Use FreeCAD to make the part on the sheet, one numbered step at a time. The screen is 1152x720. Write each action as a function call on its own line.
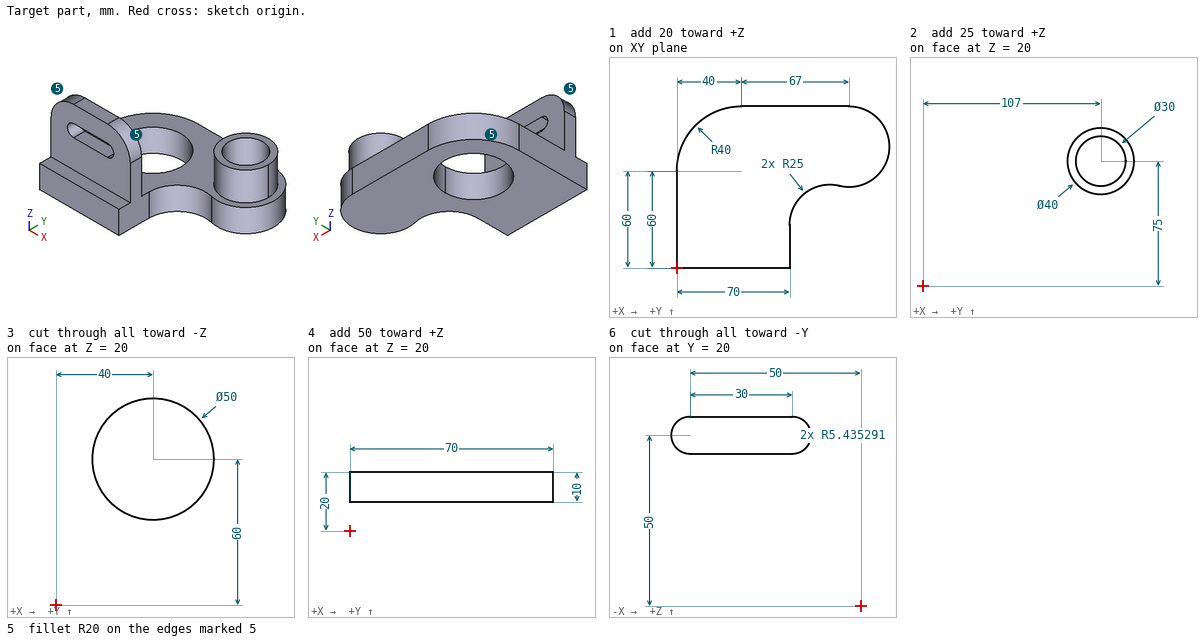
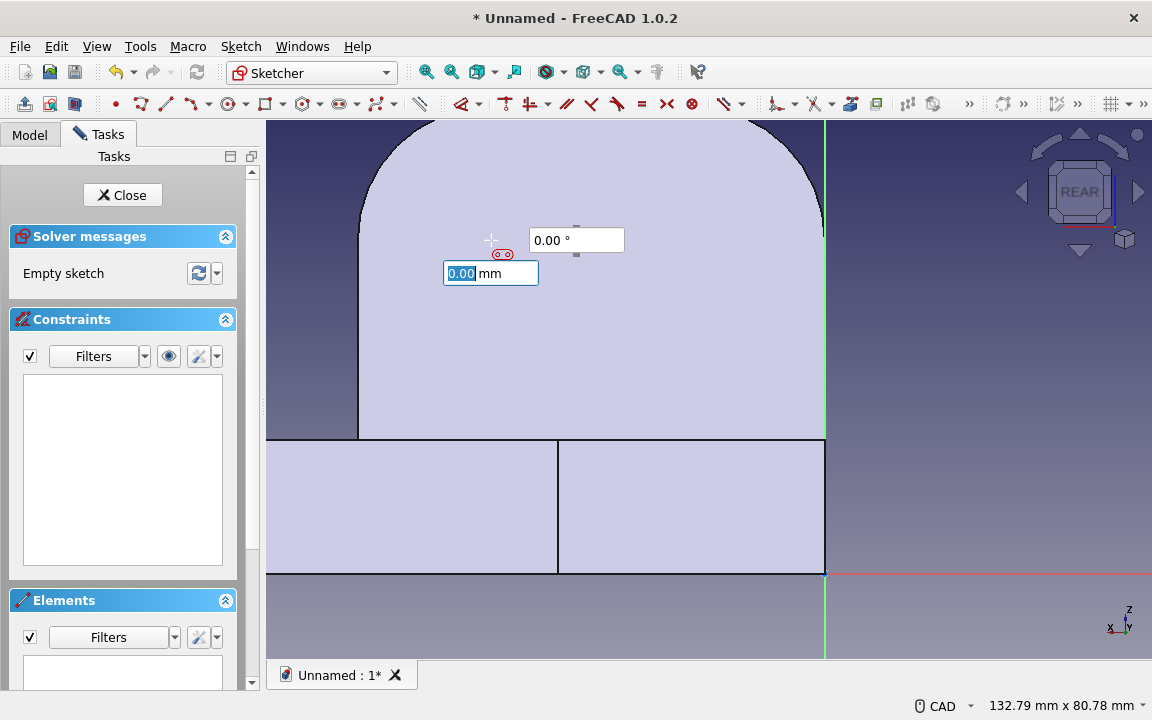
click(691, 240)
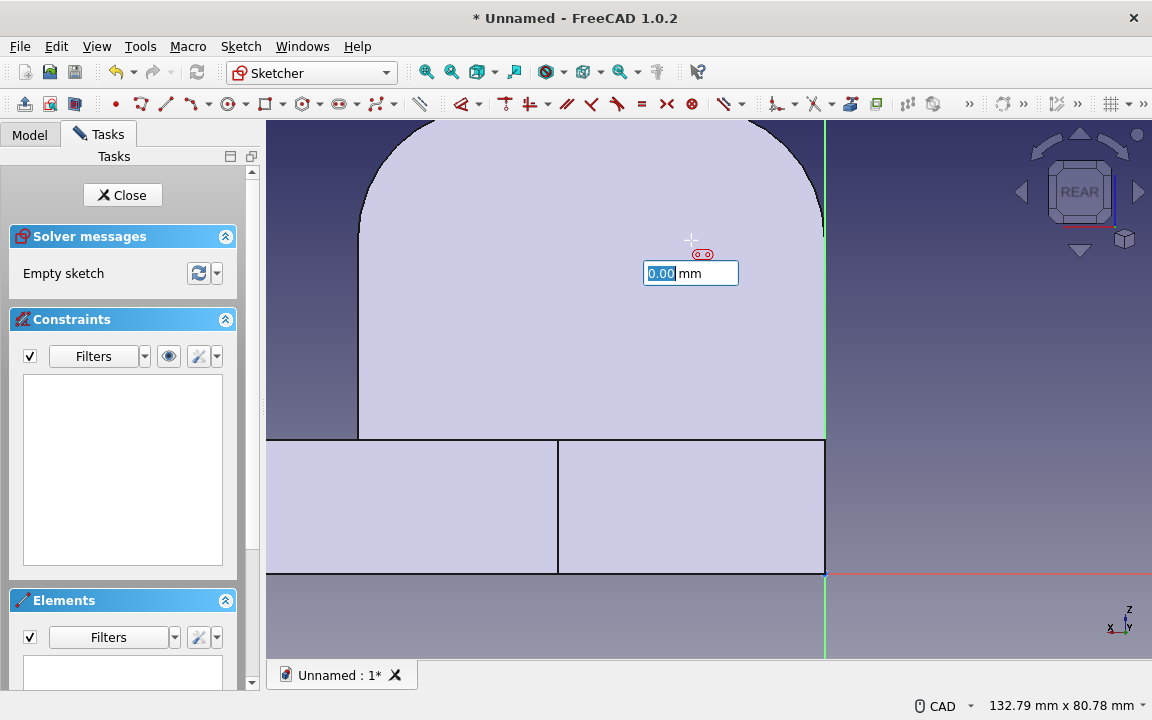
click(591, 277)
key(Escape)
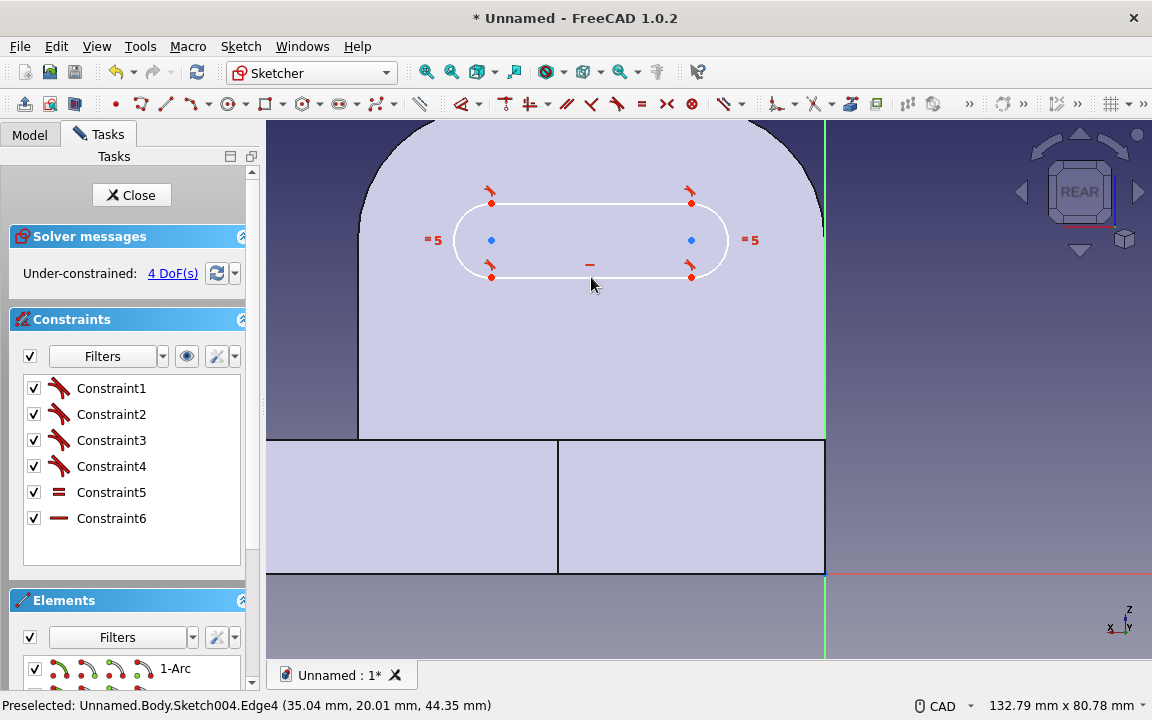
click(460, 104)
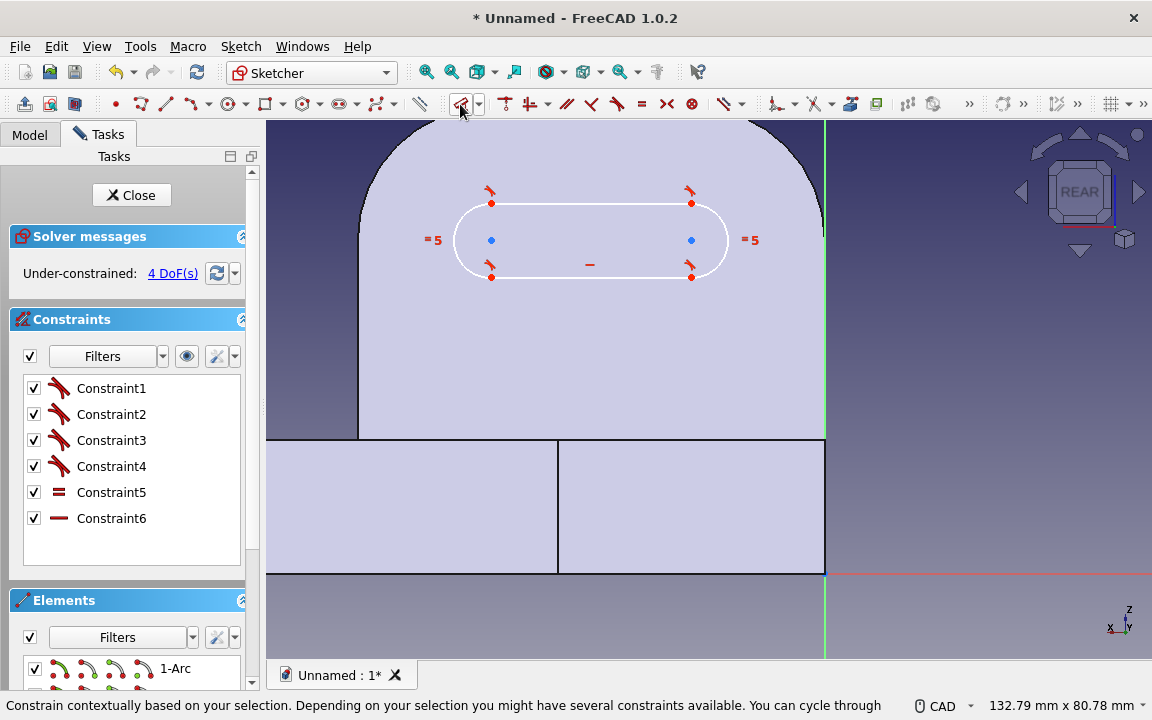
click(461, 219)
click(435, 200)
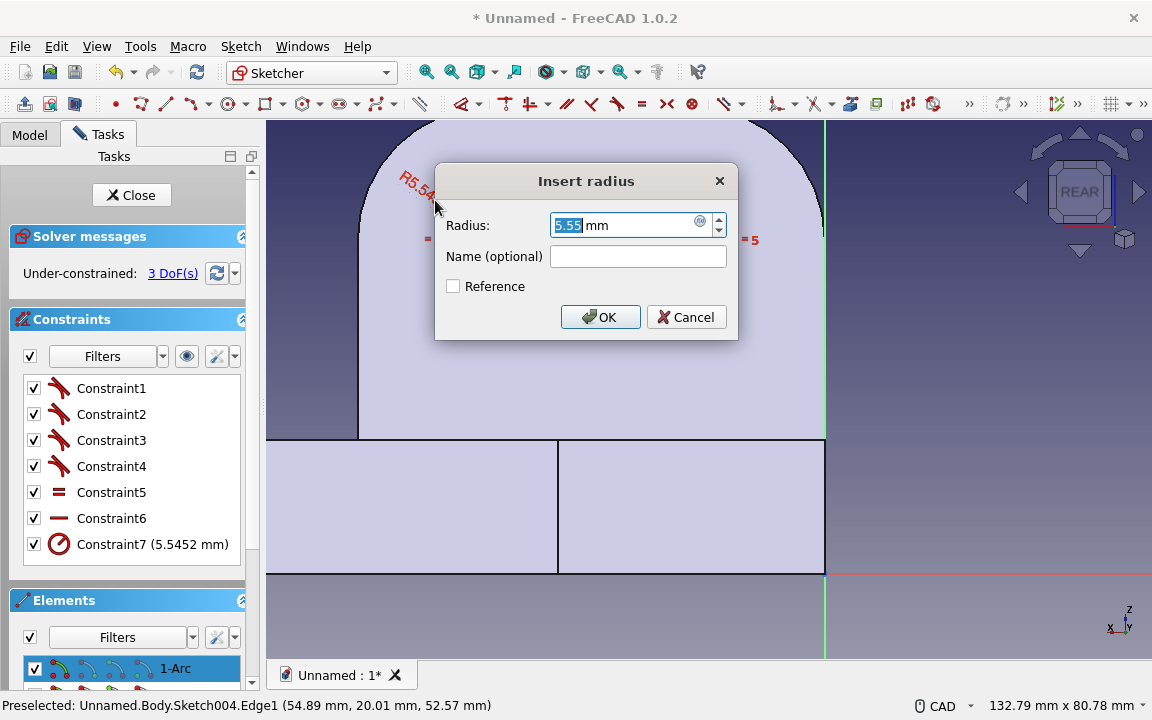
text(5.435291)
key(Return)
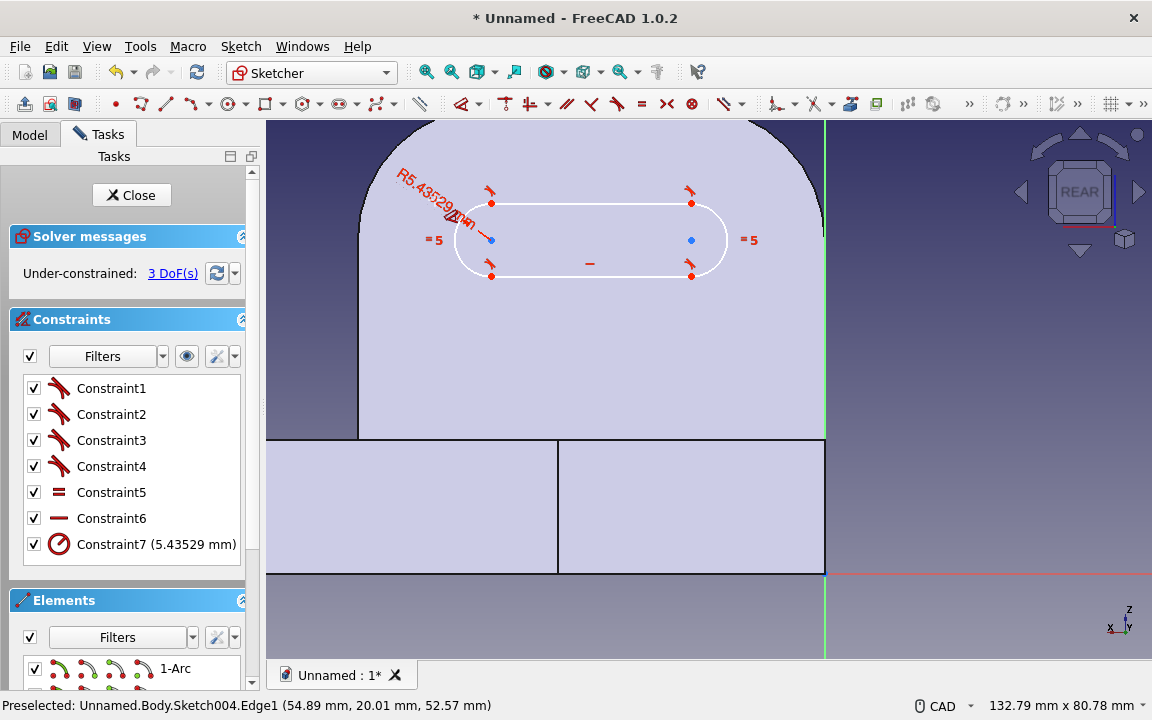
click(551, 204)
click(591, 170)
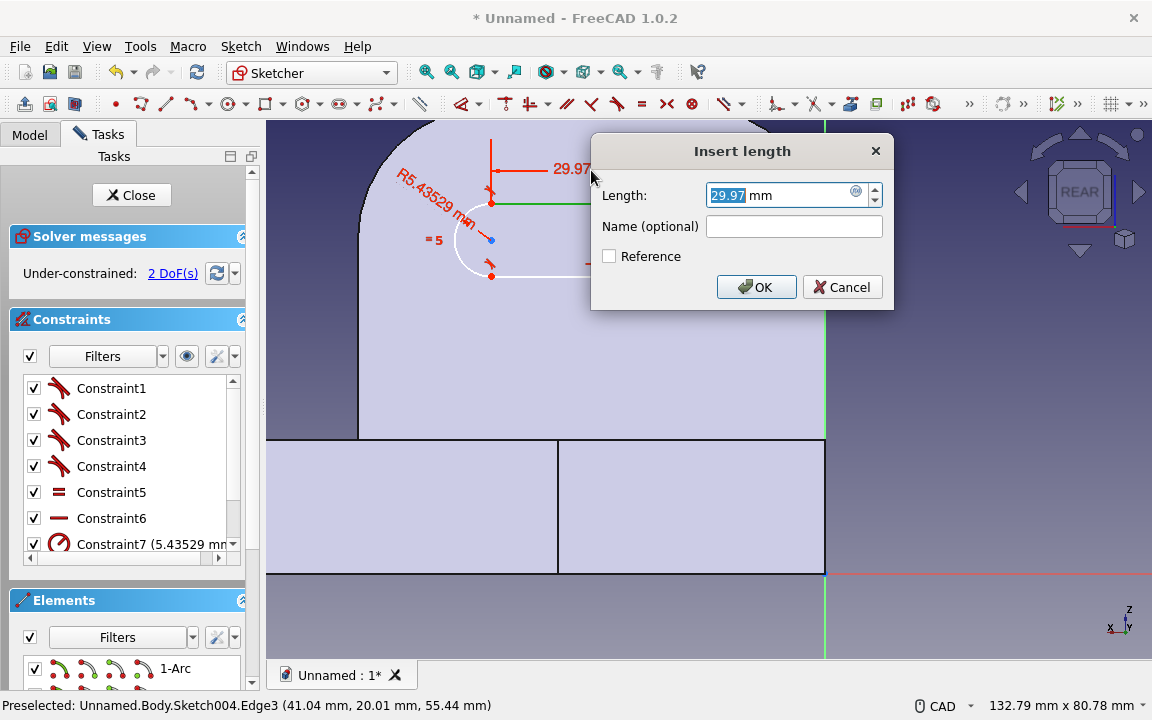
text(30)
key(Return)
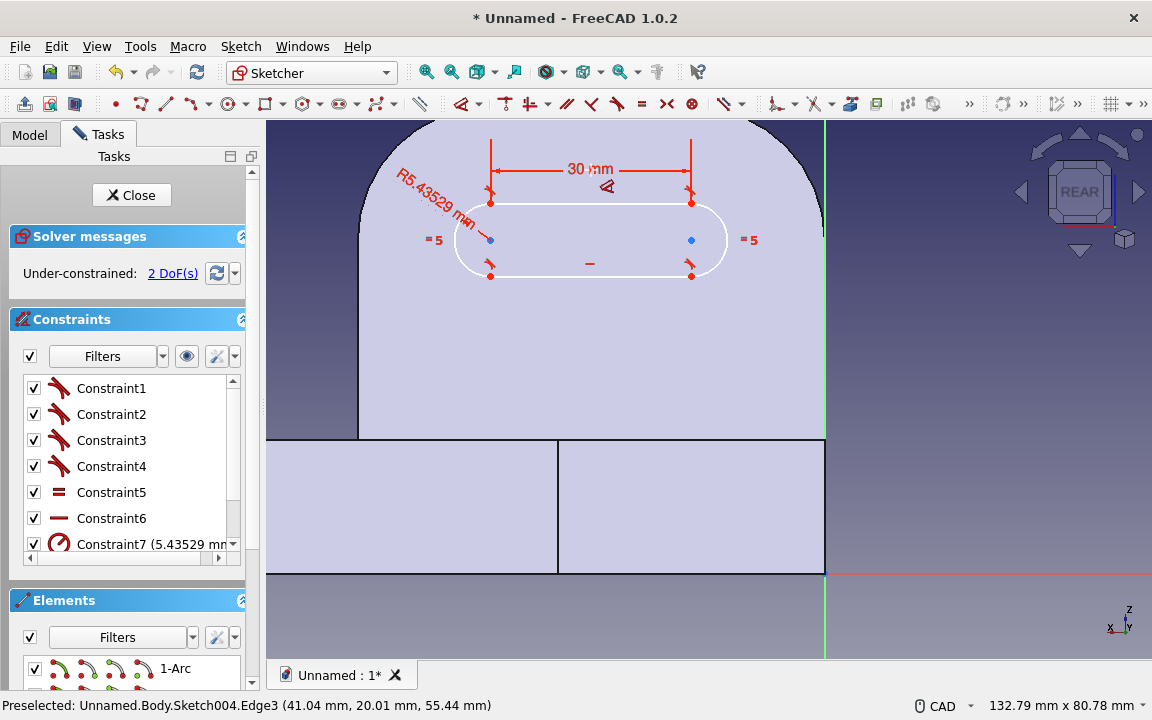
click(491, 204)
click(735, 170)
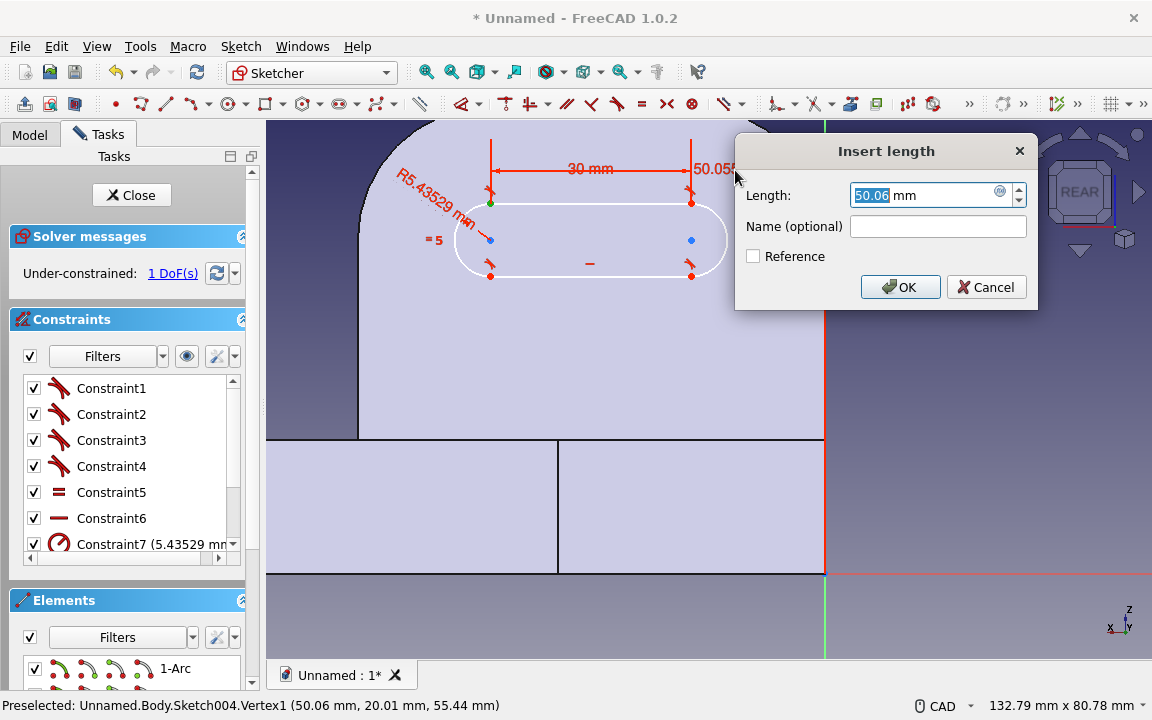
text(50)
key(Return)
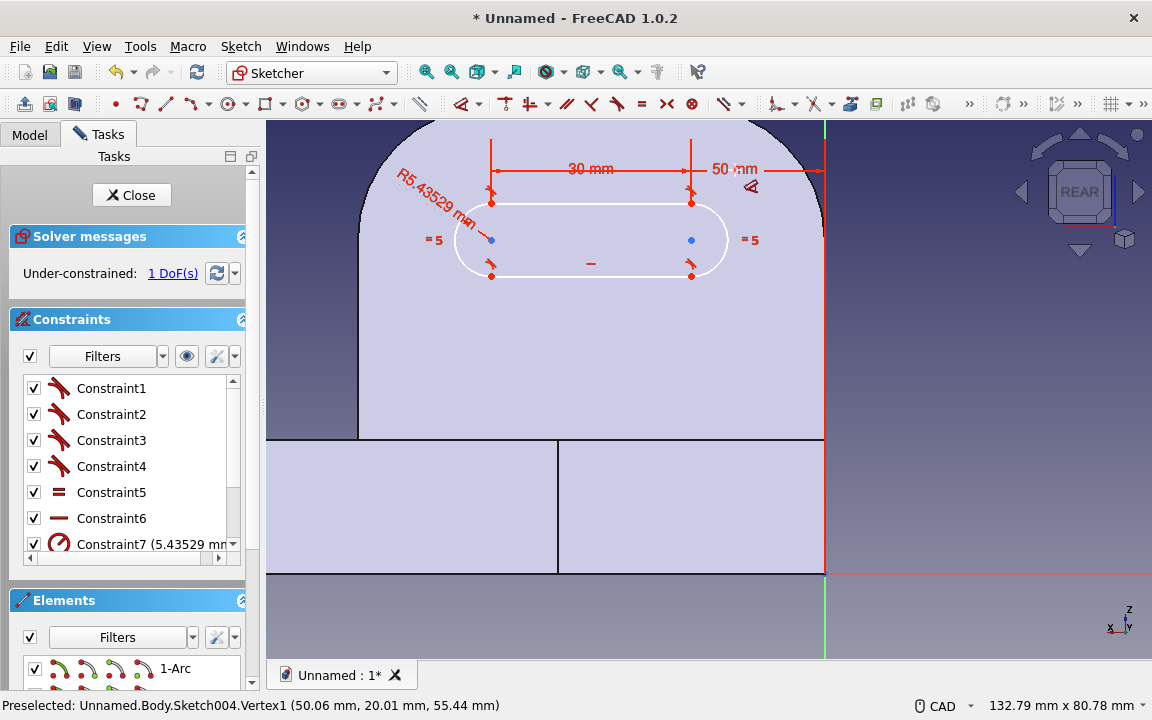
click(491, 240)
click(859, 407)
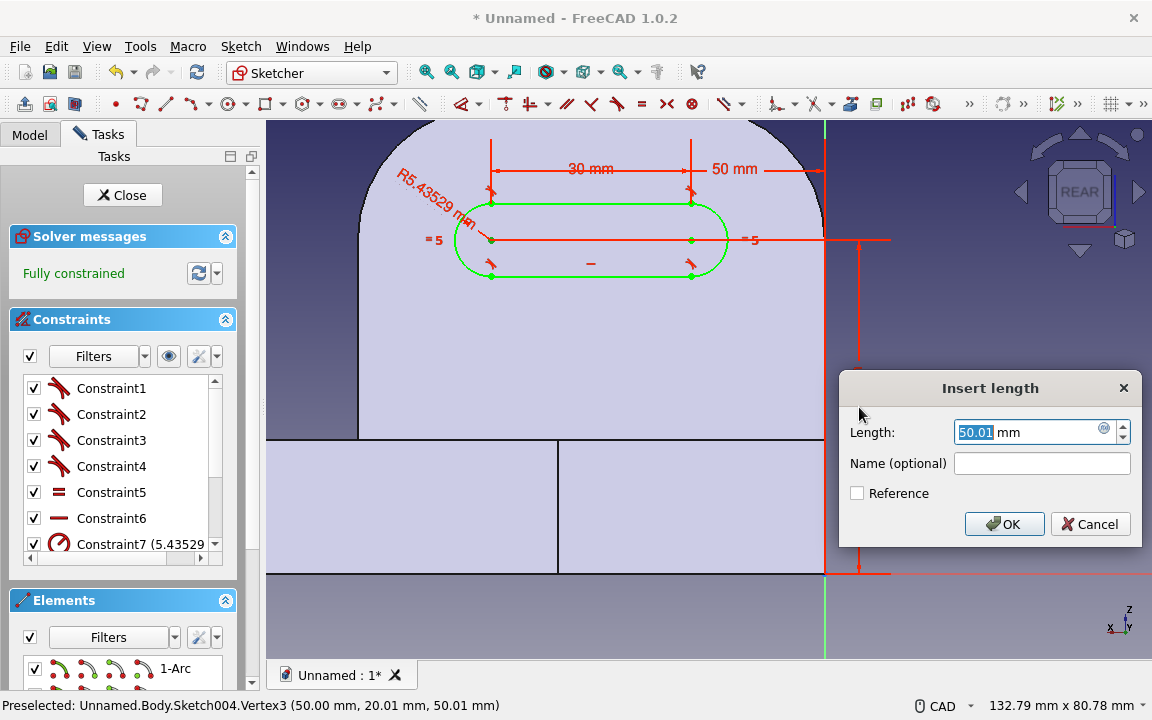
text(50)
key(Return)
key(Escape)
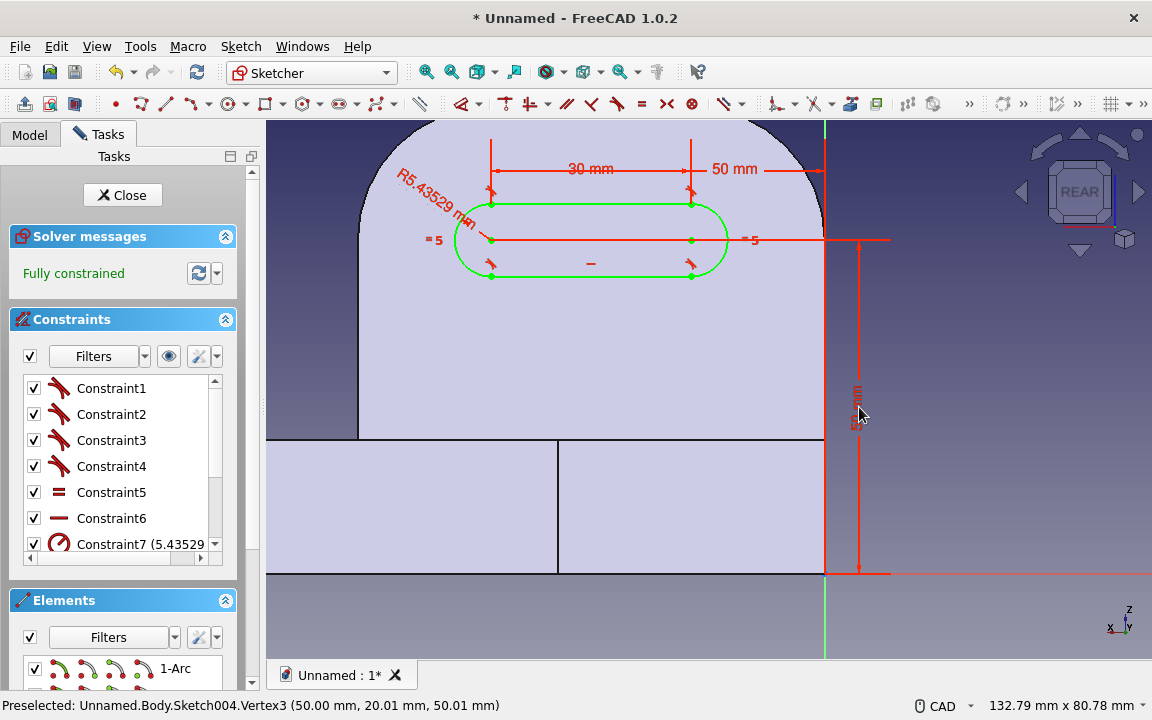
click(123, 195)